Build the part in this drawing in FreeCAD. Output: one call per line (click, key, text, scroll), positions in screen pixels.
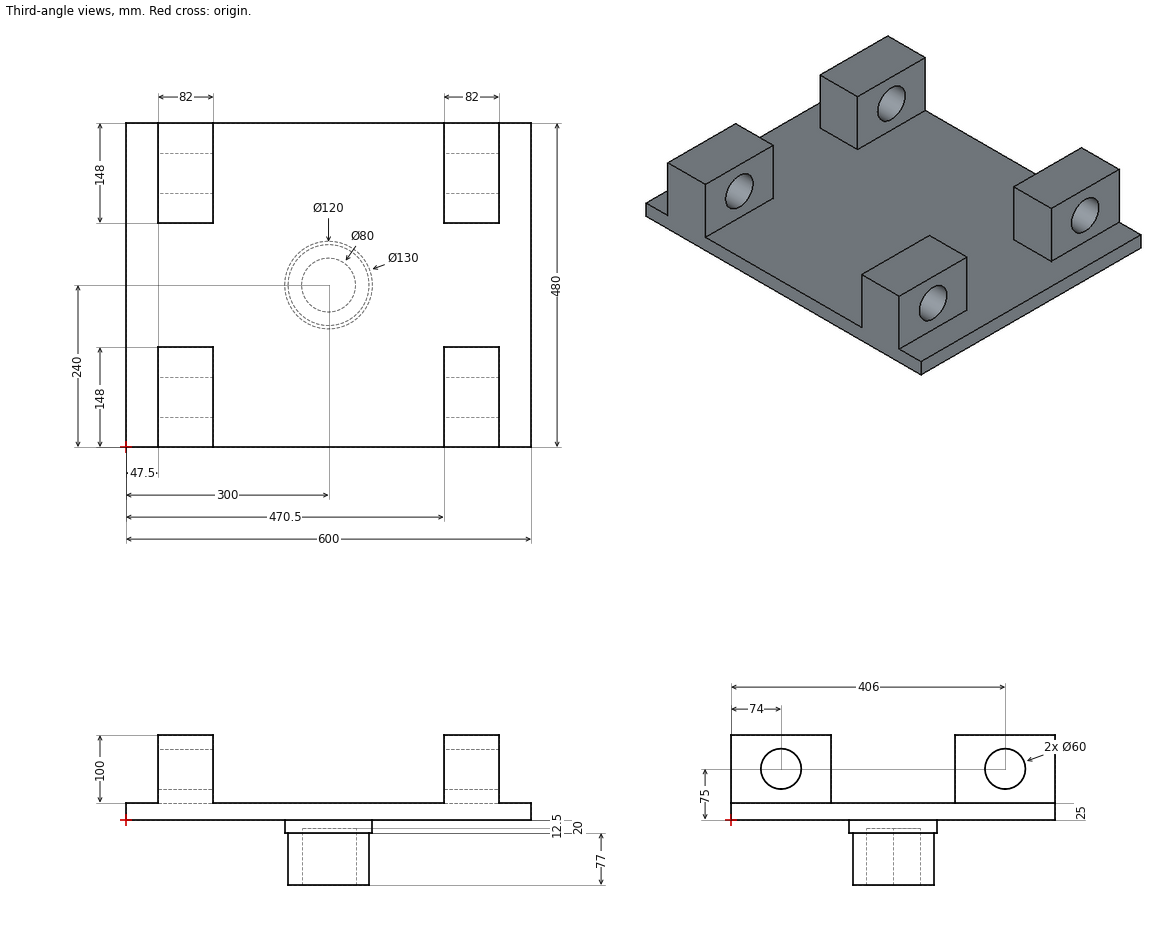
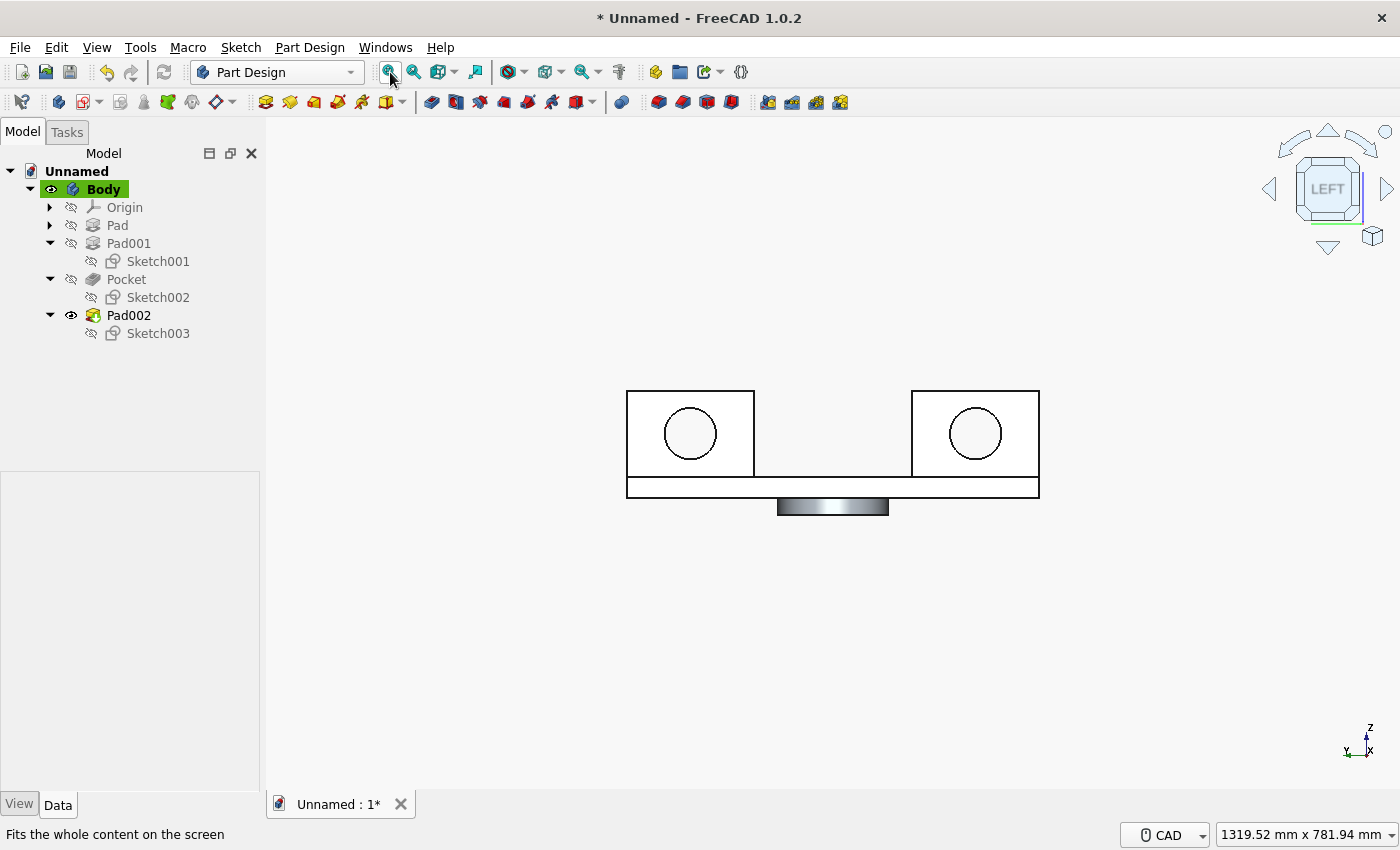
key(5)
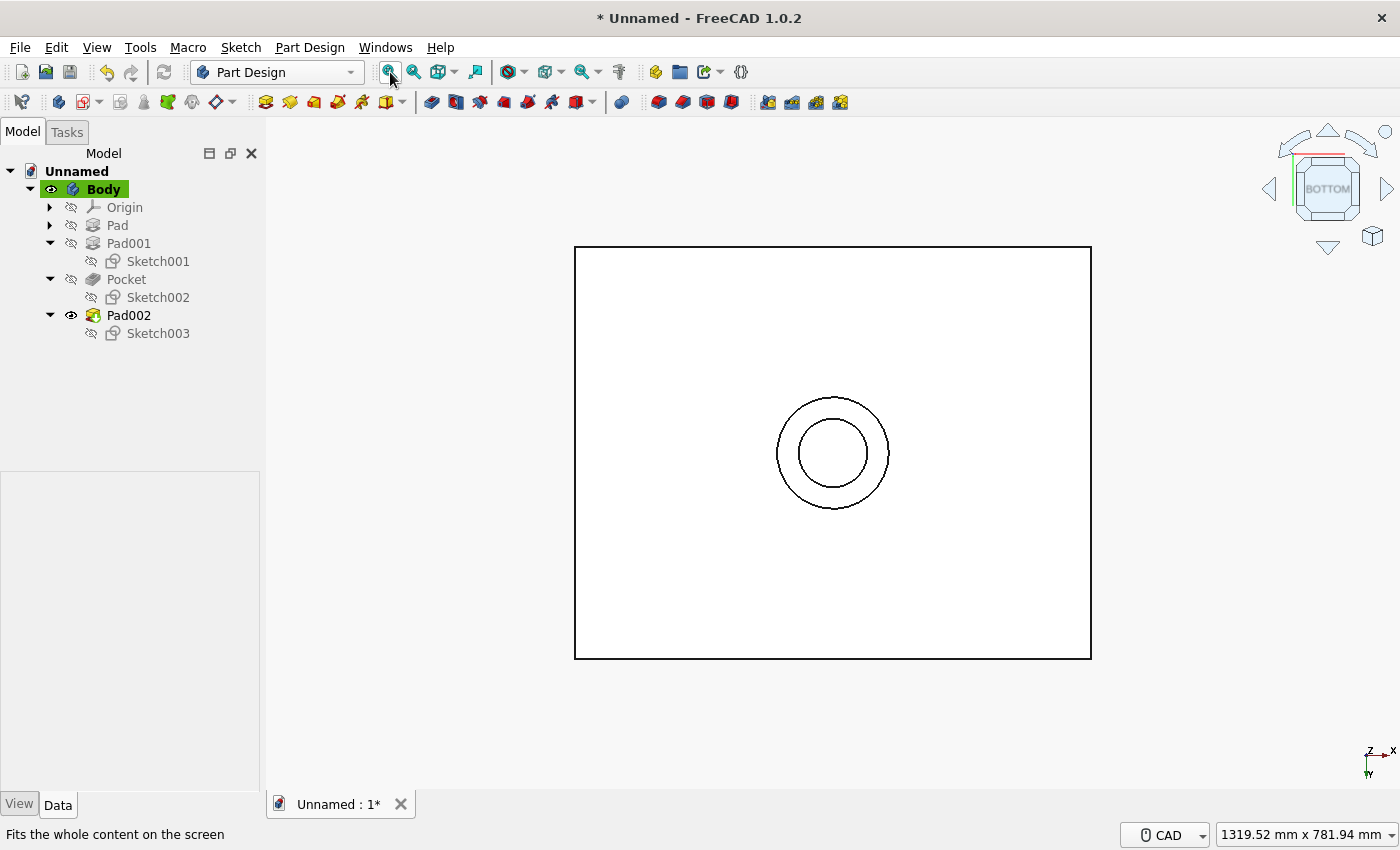
click(801, 484)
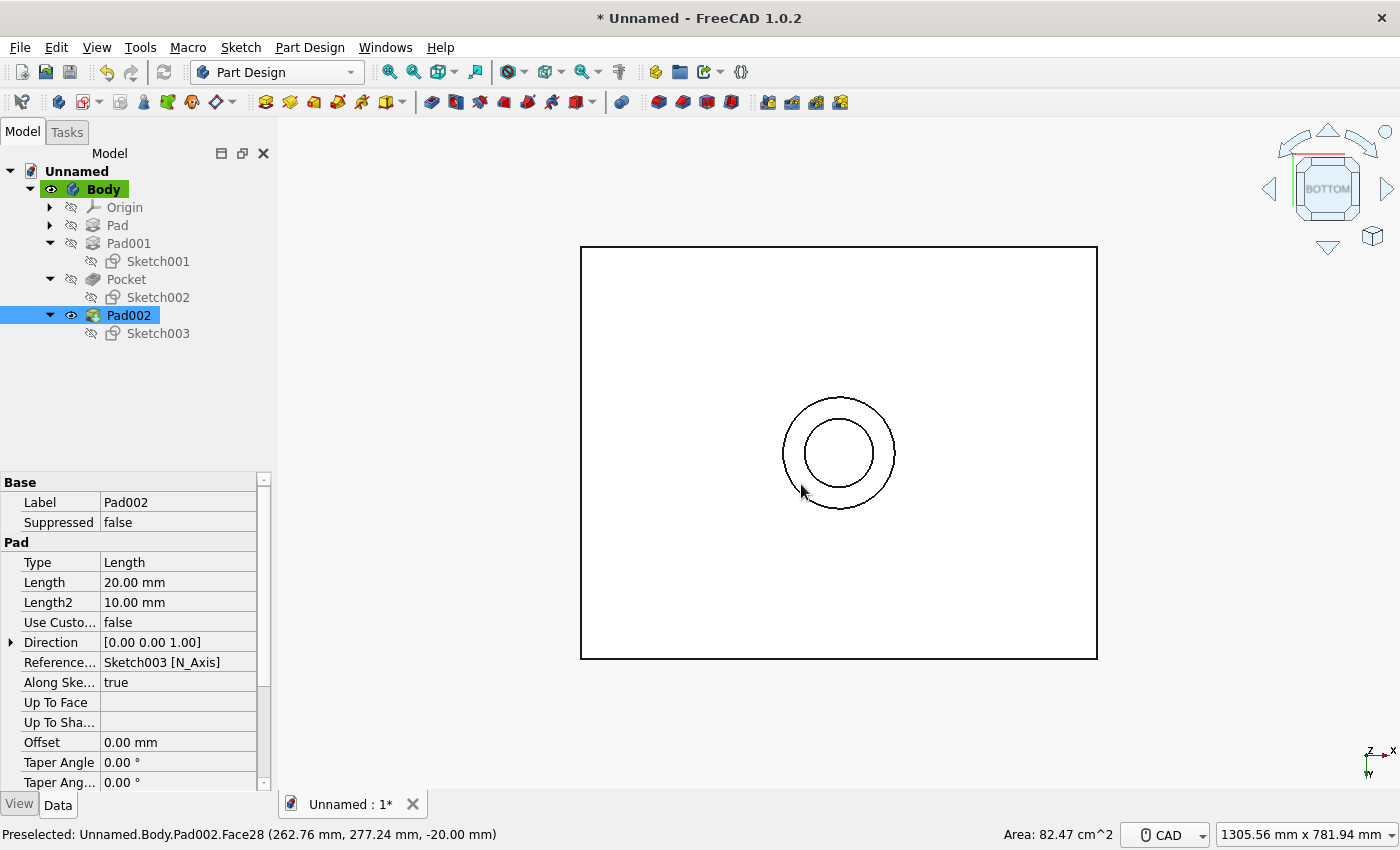
click(84, 102)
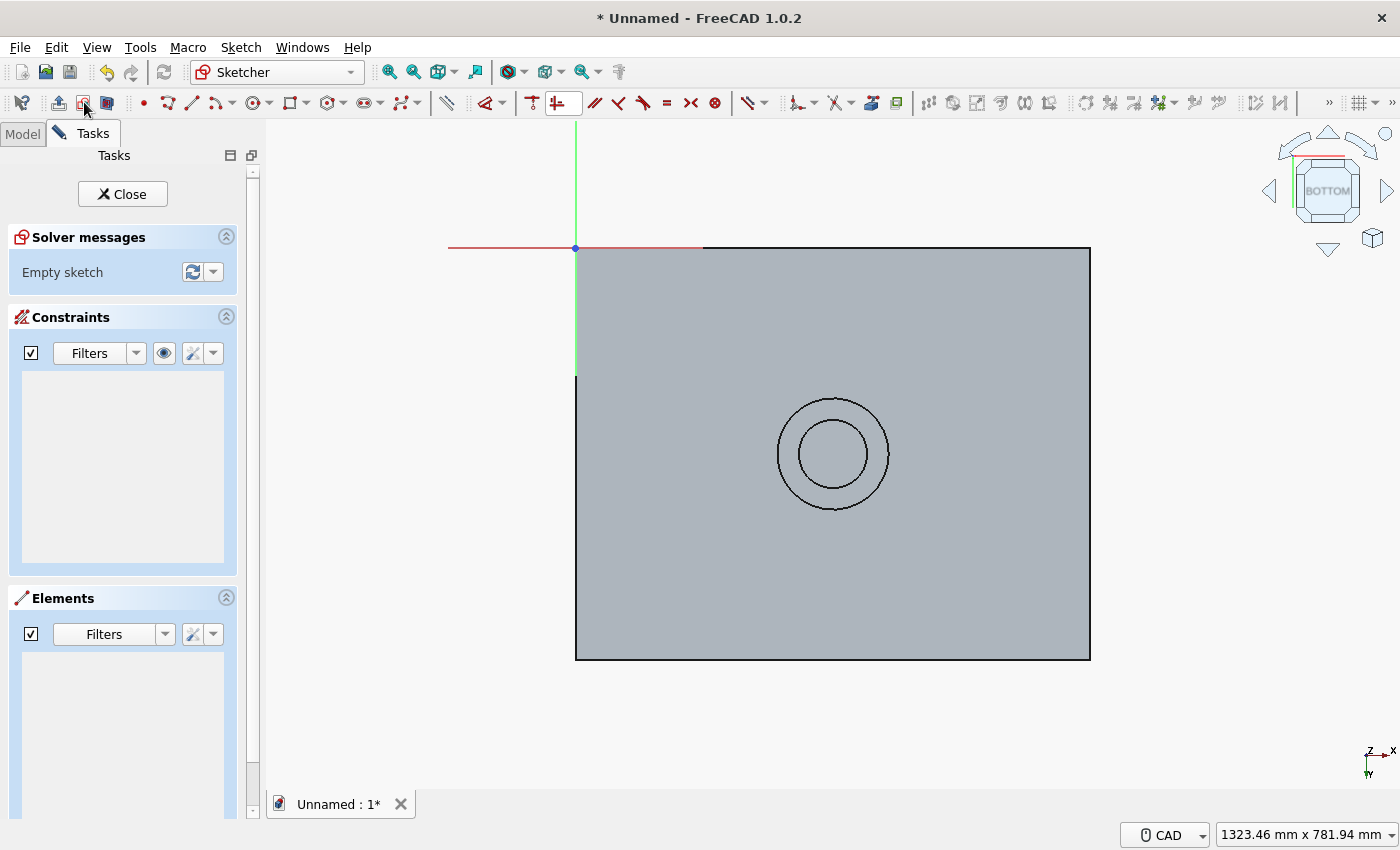
scroll(855, 454, up, 7)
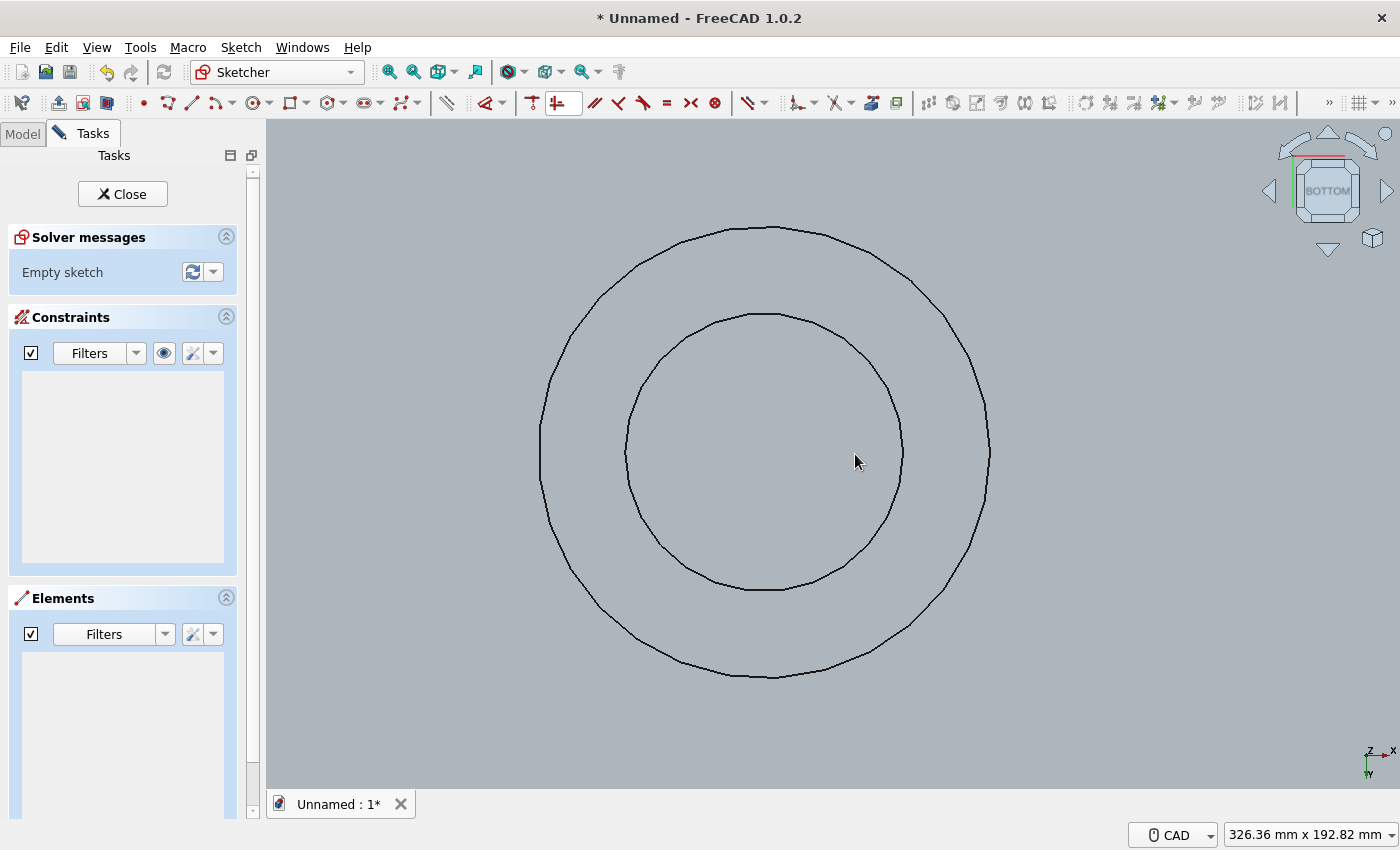
click(254, 104)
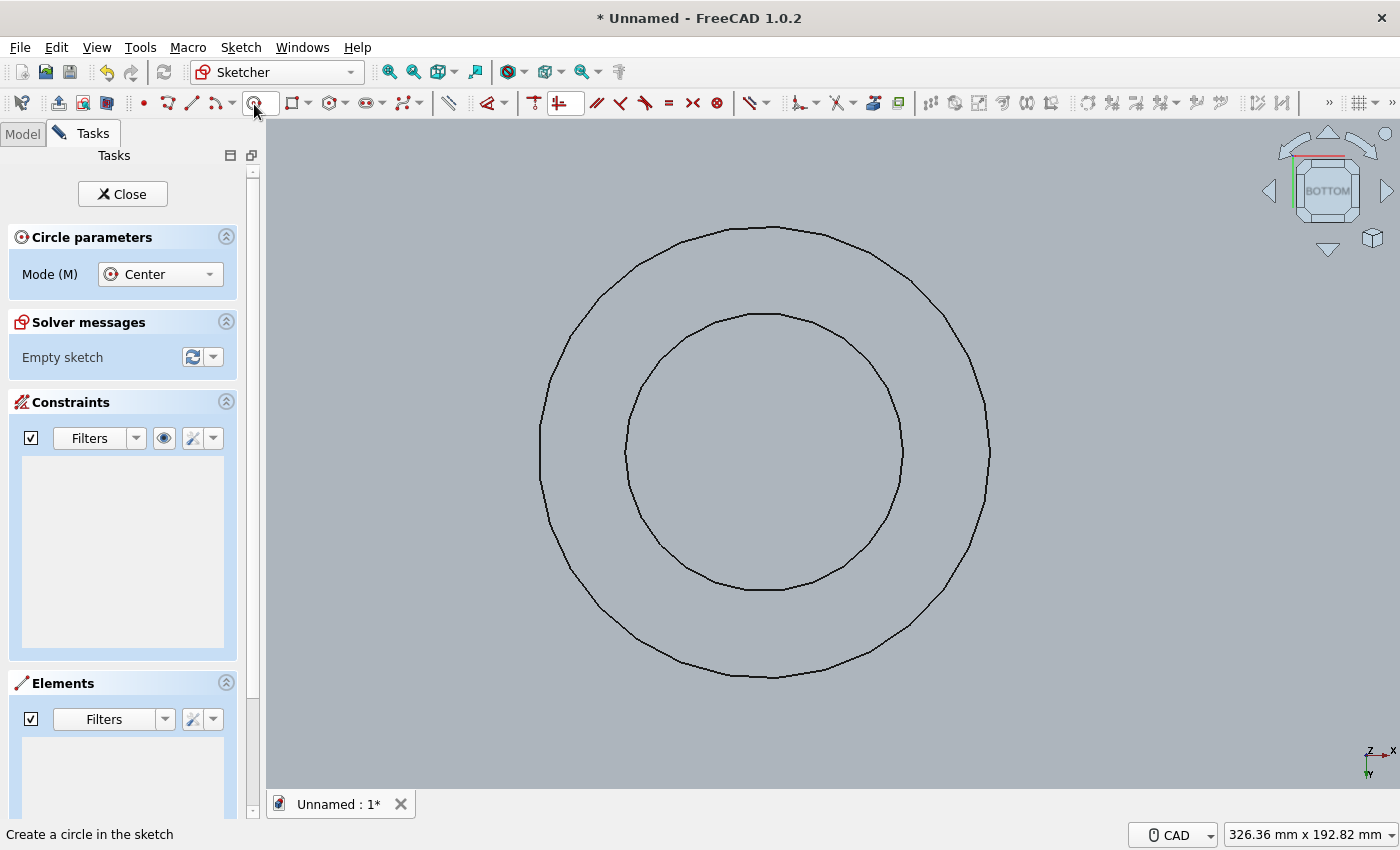
click(764, 452)
move(912, 305)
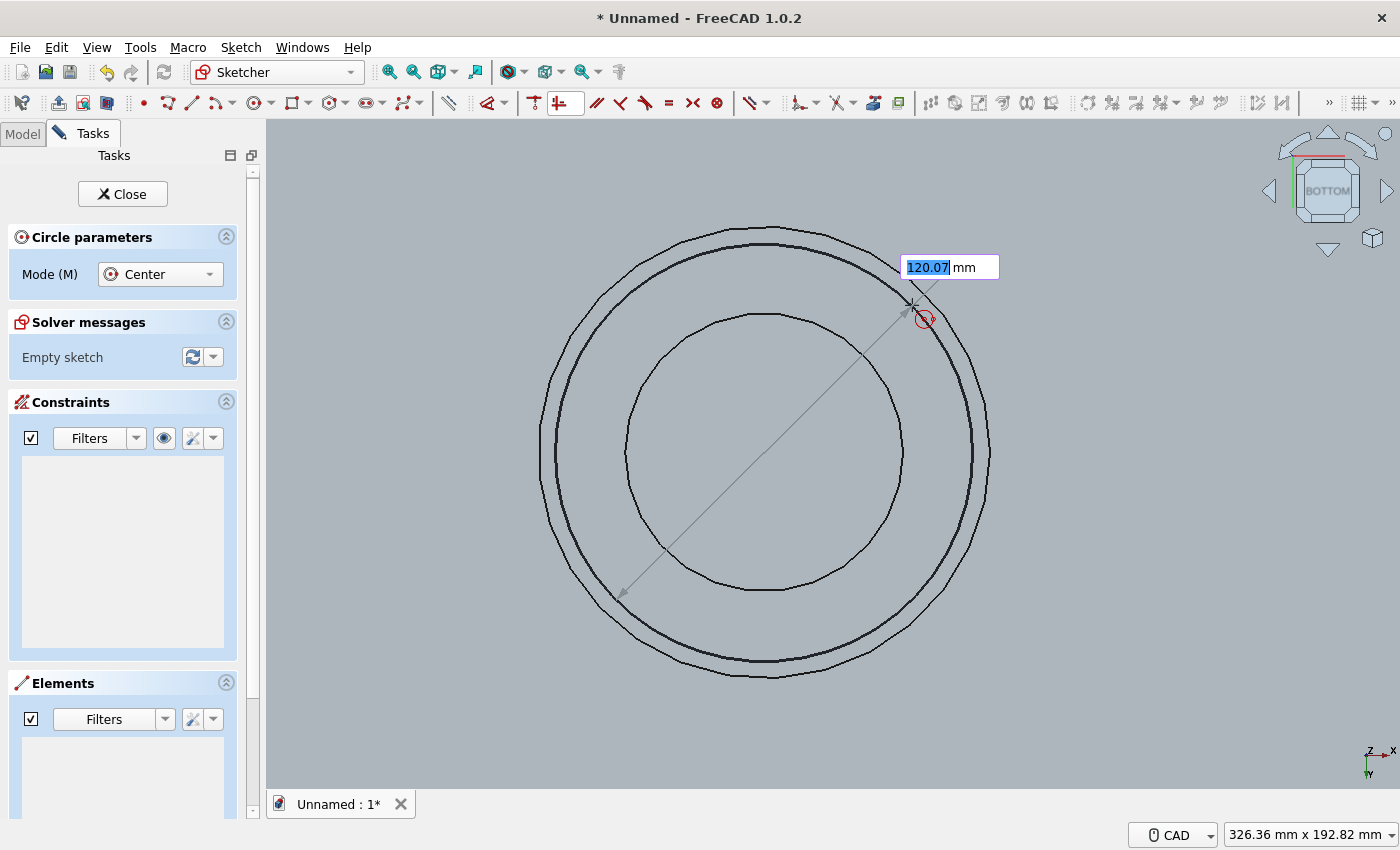
text(120)
key(Return)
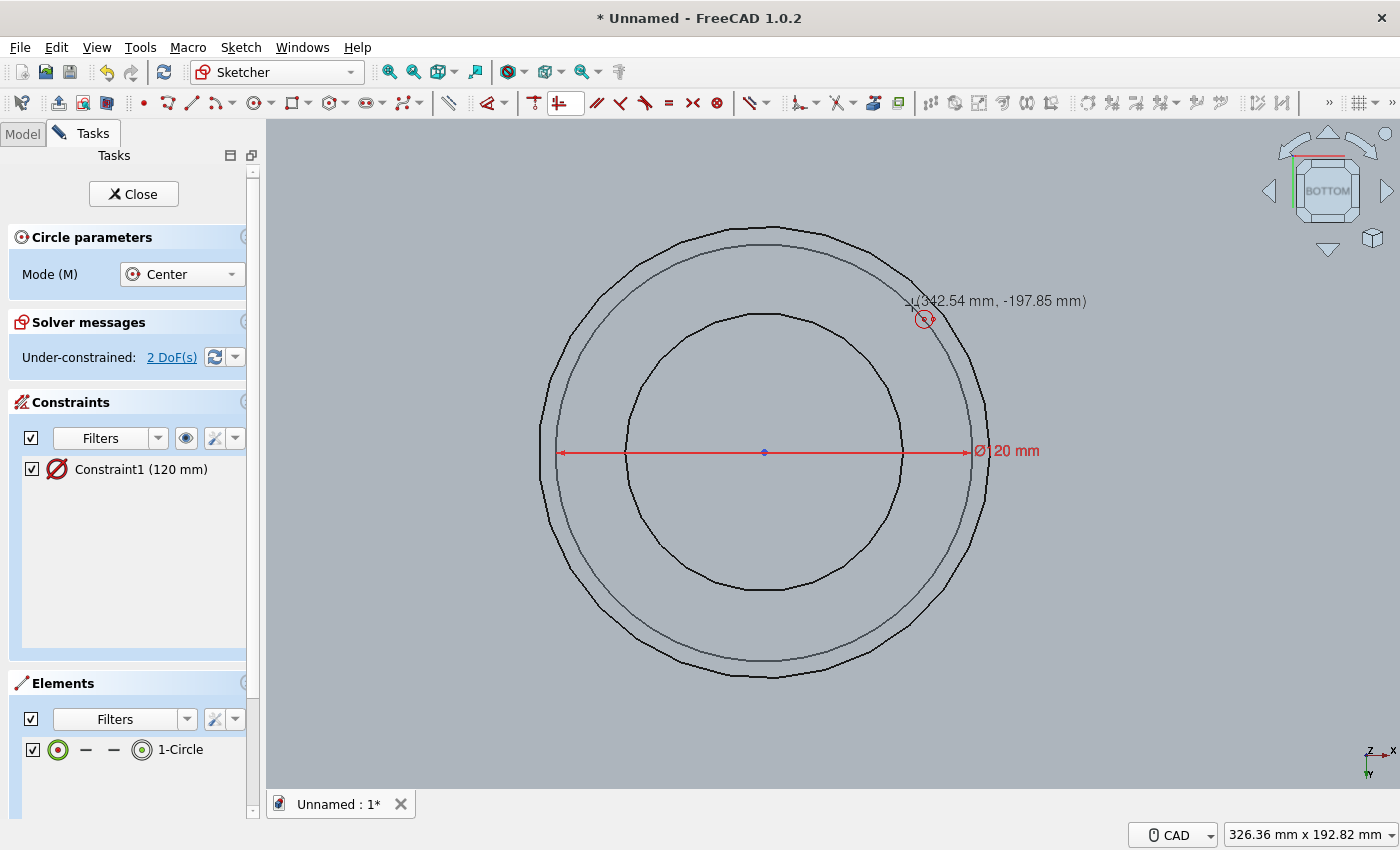
click(764, 453)
move(862, 354)